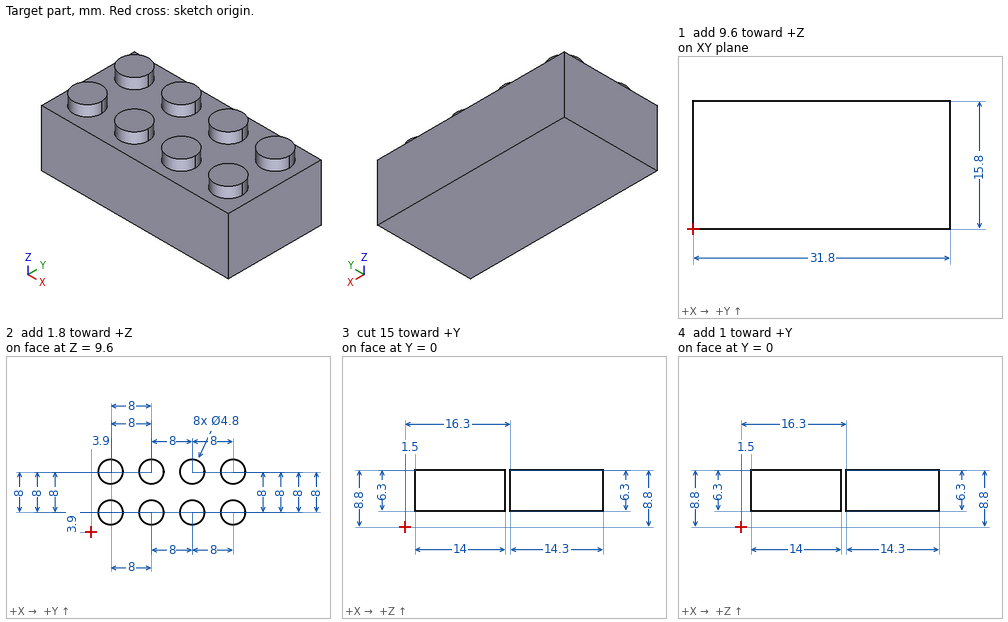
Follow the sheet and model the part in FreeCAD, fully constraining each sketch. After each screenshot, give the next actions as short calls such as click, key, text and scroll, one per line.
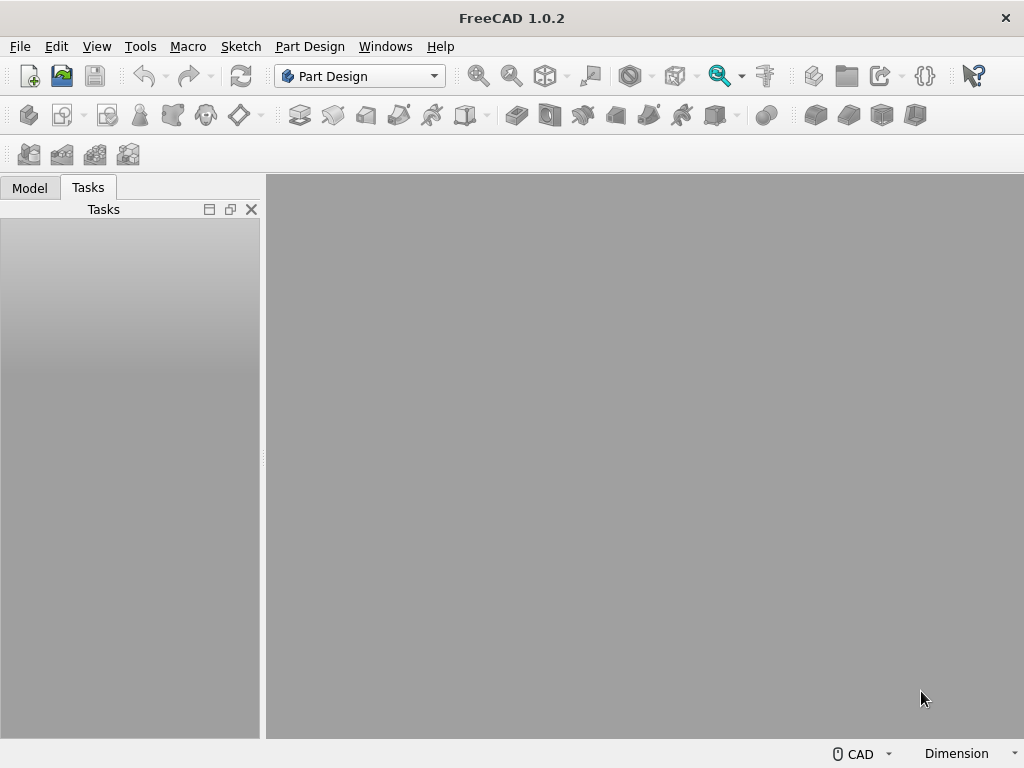
key(ctrl+n)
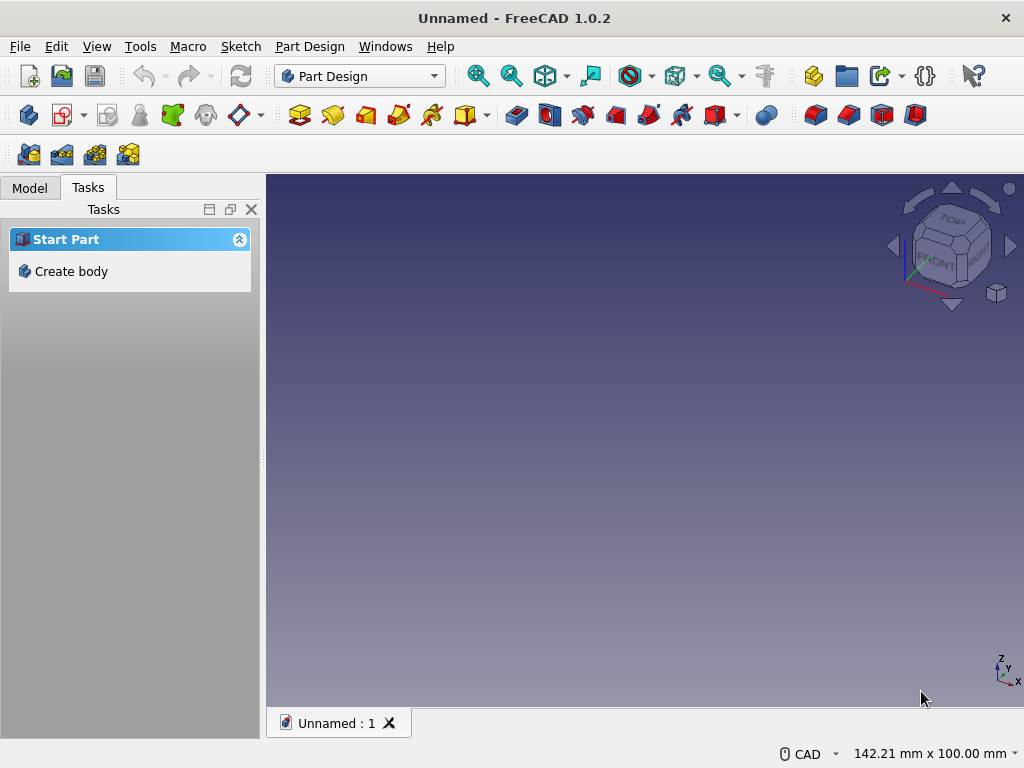
click(62, 116)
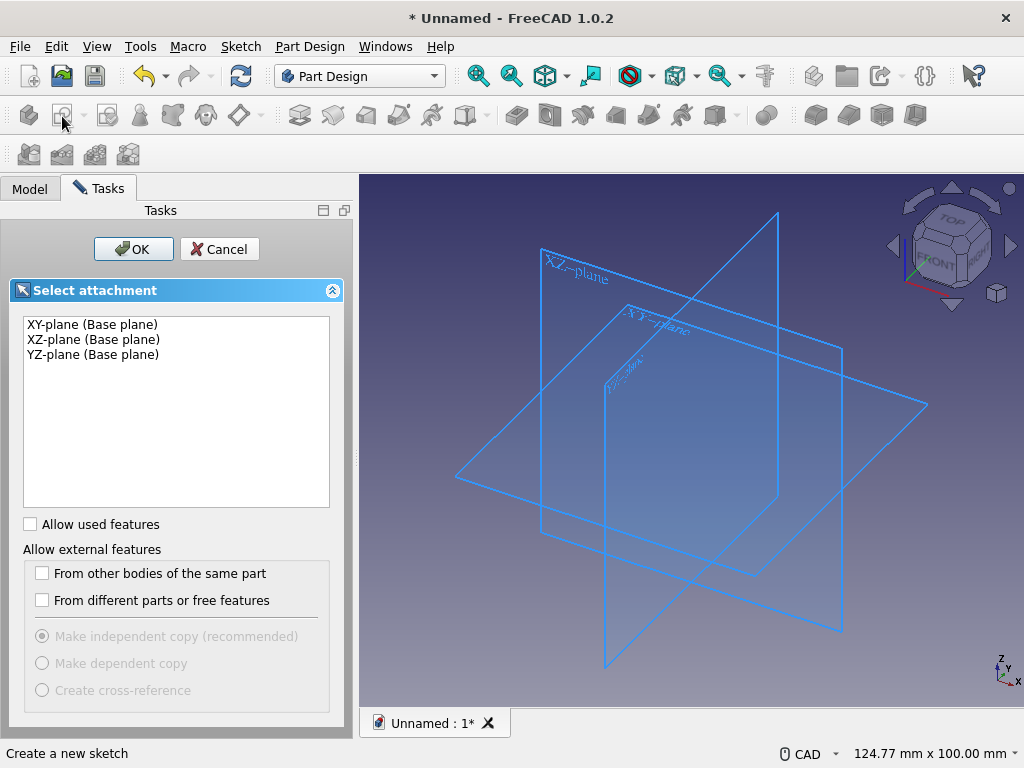
click(84, 324)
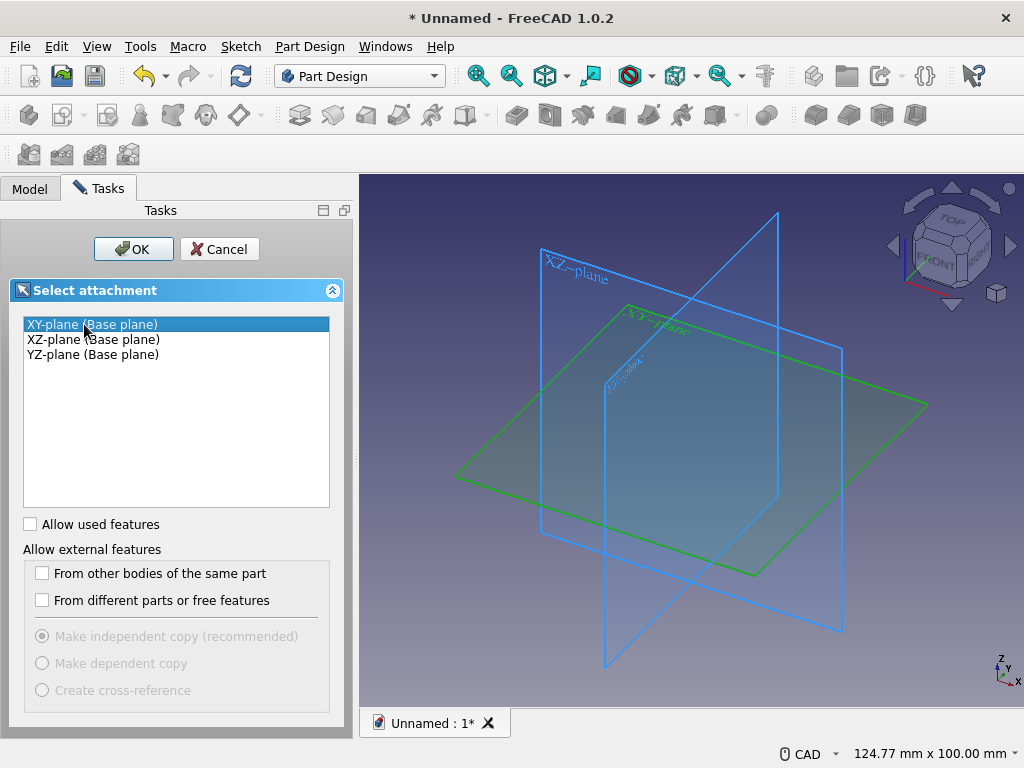
click(134, 249)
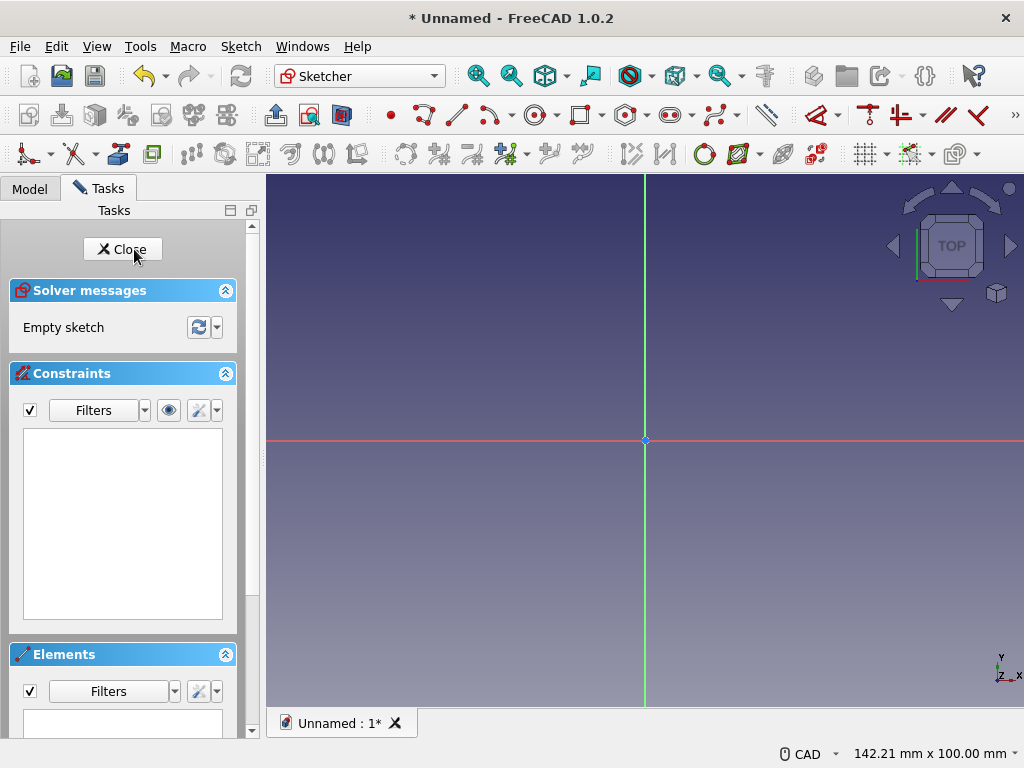
scroll(855, 364, up, 4)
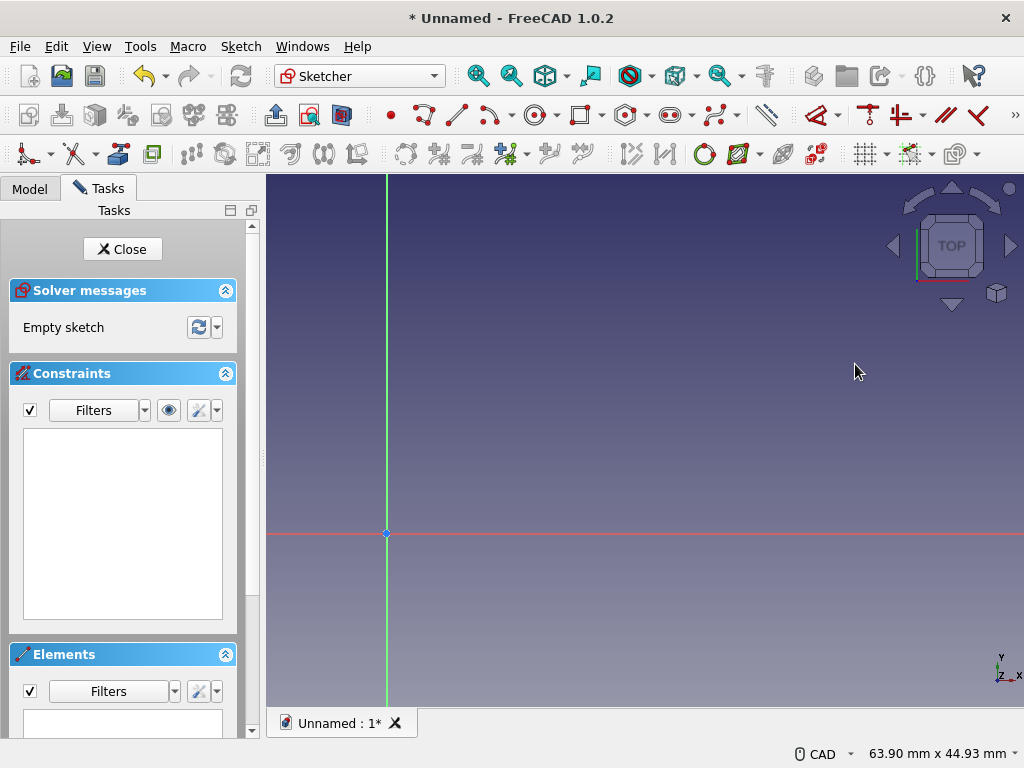
click(580, 116)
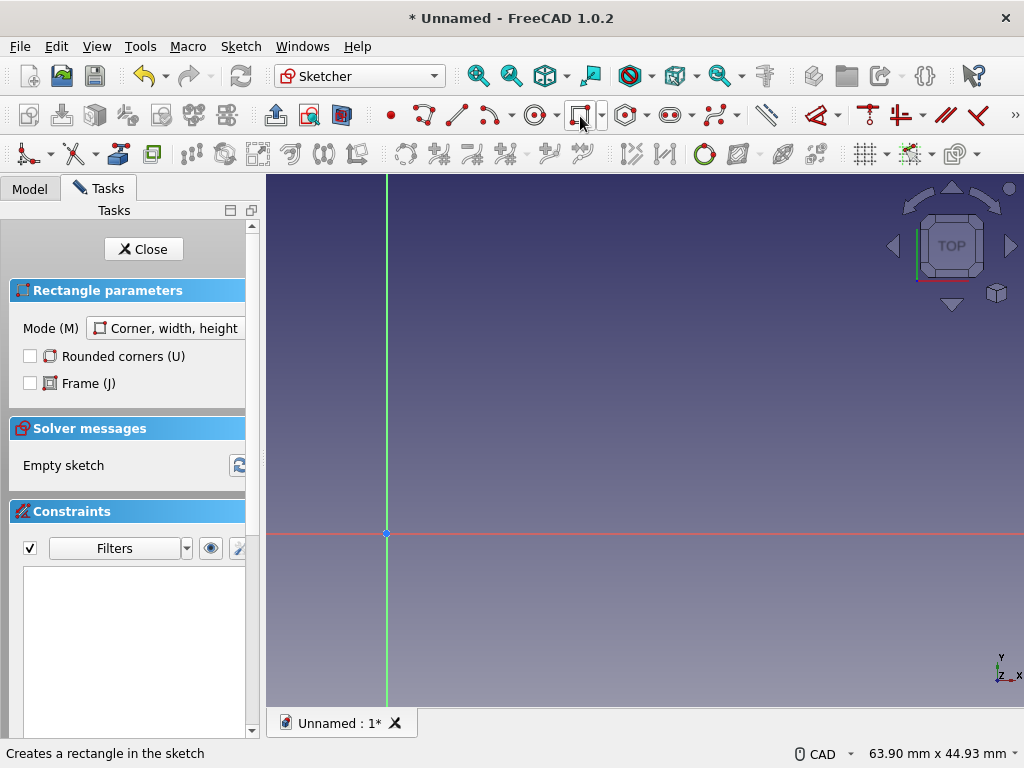
click(387, 534)
click(764, 346)
key(Escape)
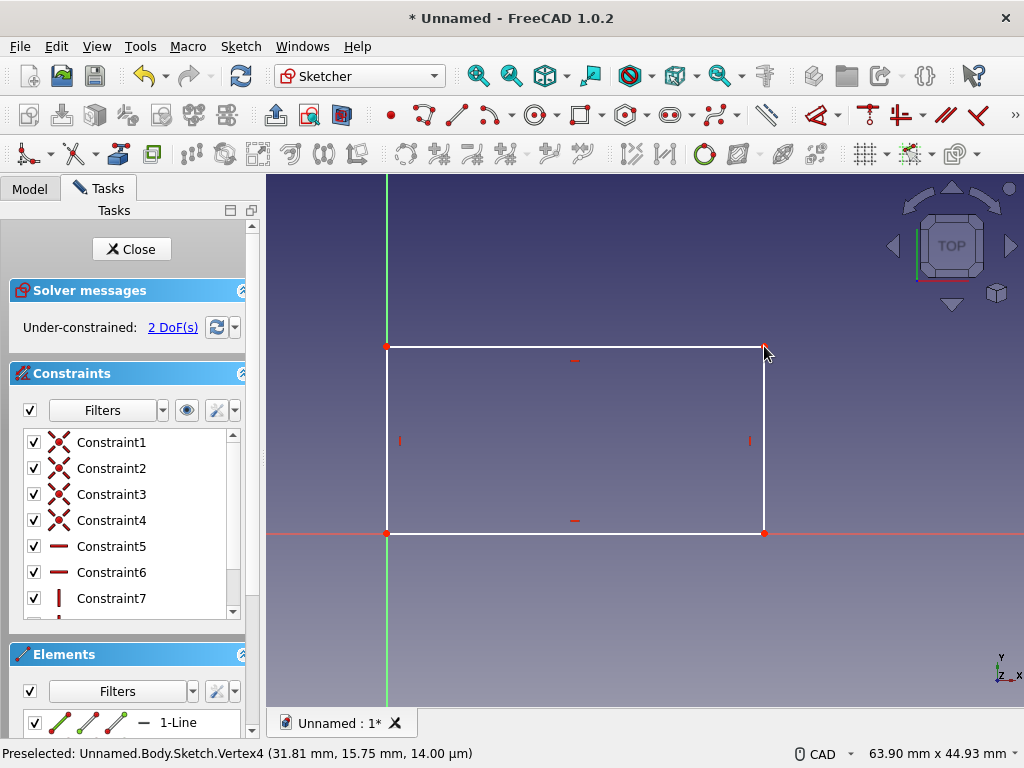
key(d)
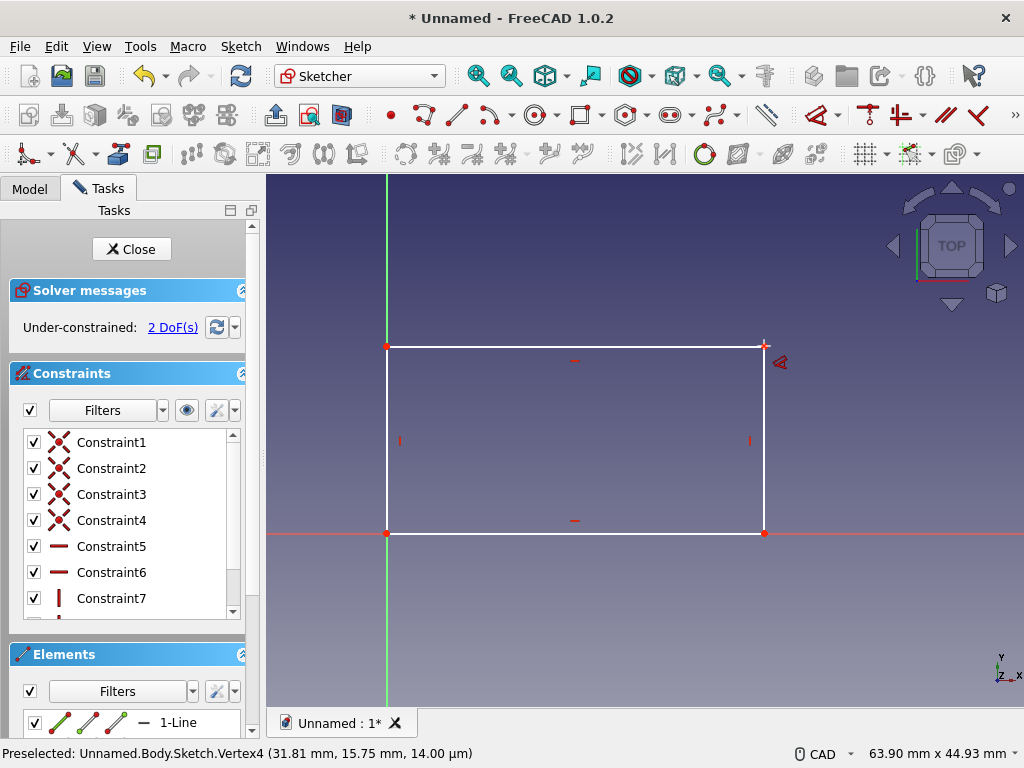
click(500, 534)
click(575, 568)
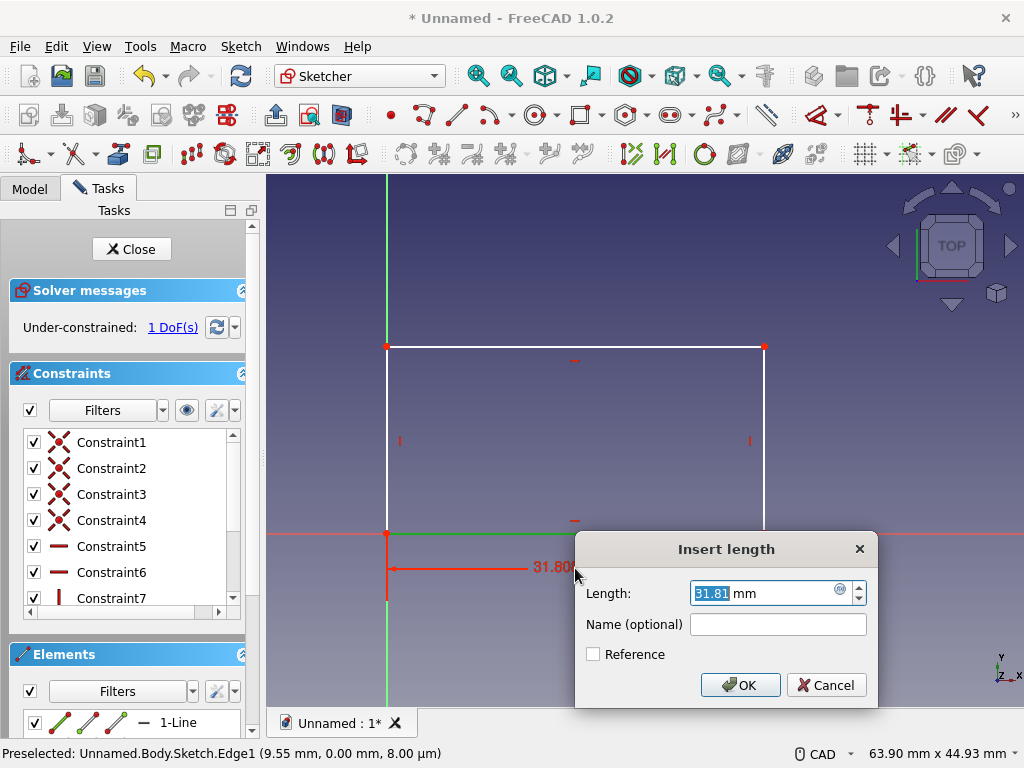
text(31.8)
key(Return)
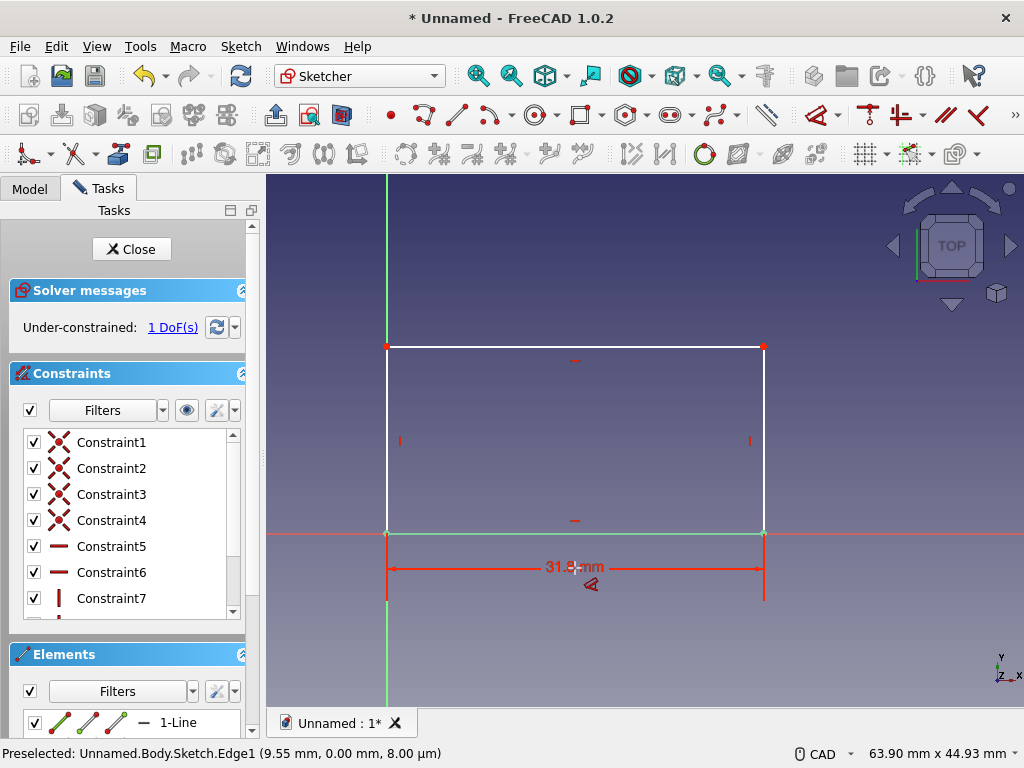
click(764, 478)
click(798, 440)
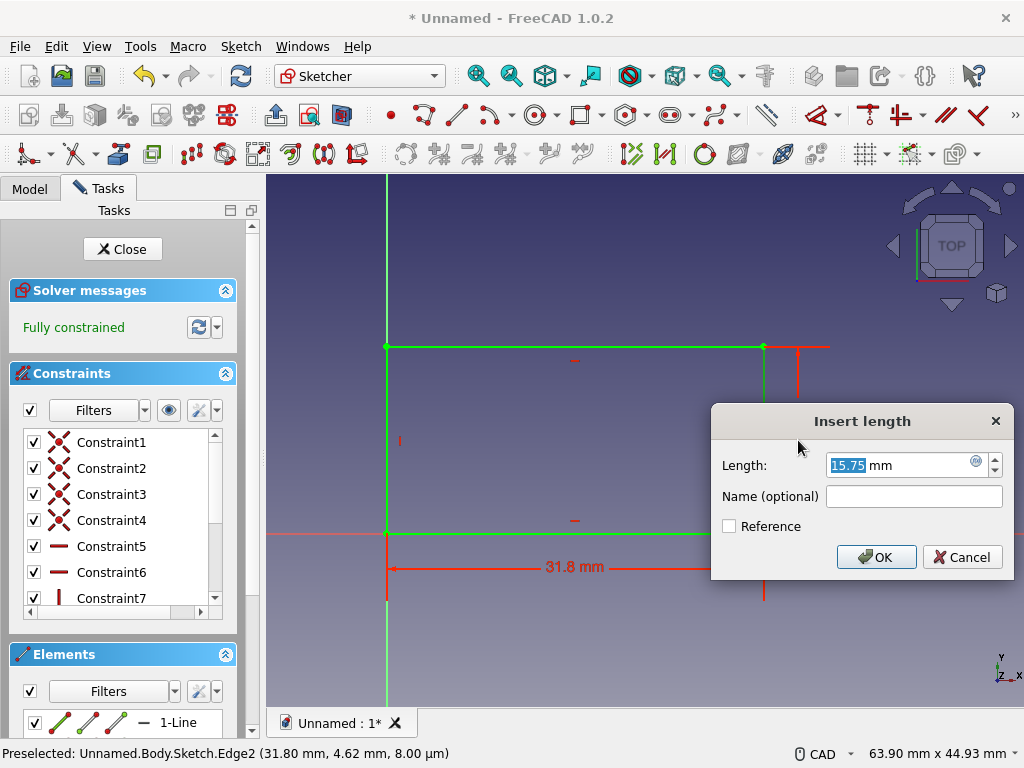
text(15.8)
key(Return)
key(Escape)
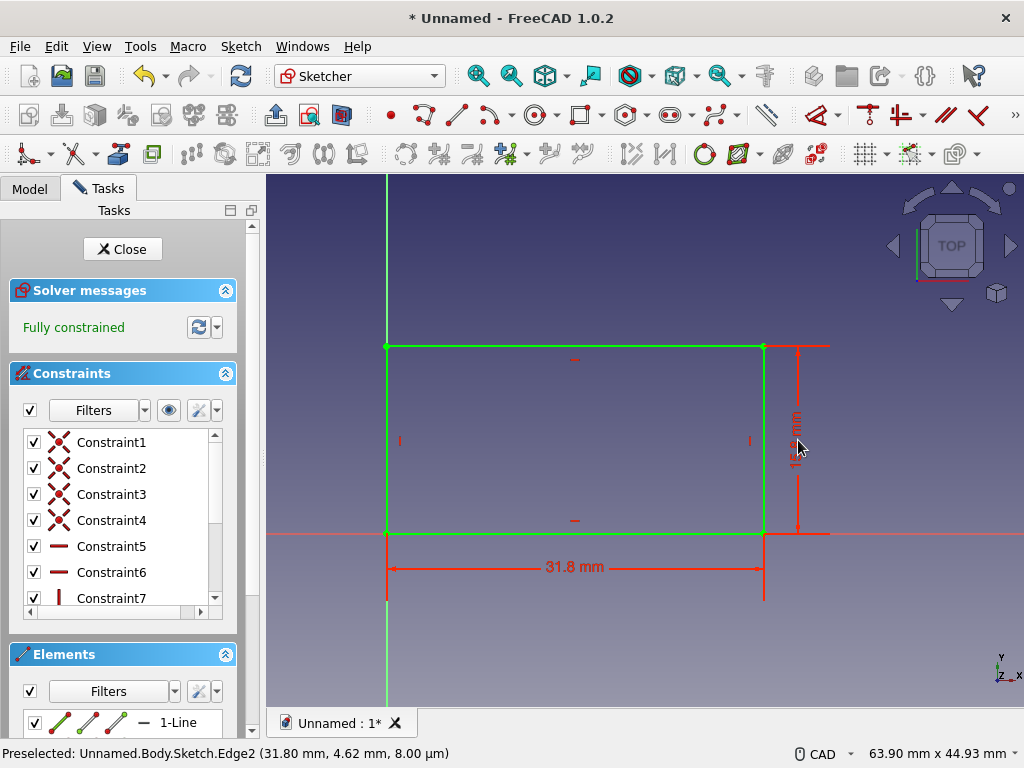
click(123, 249)